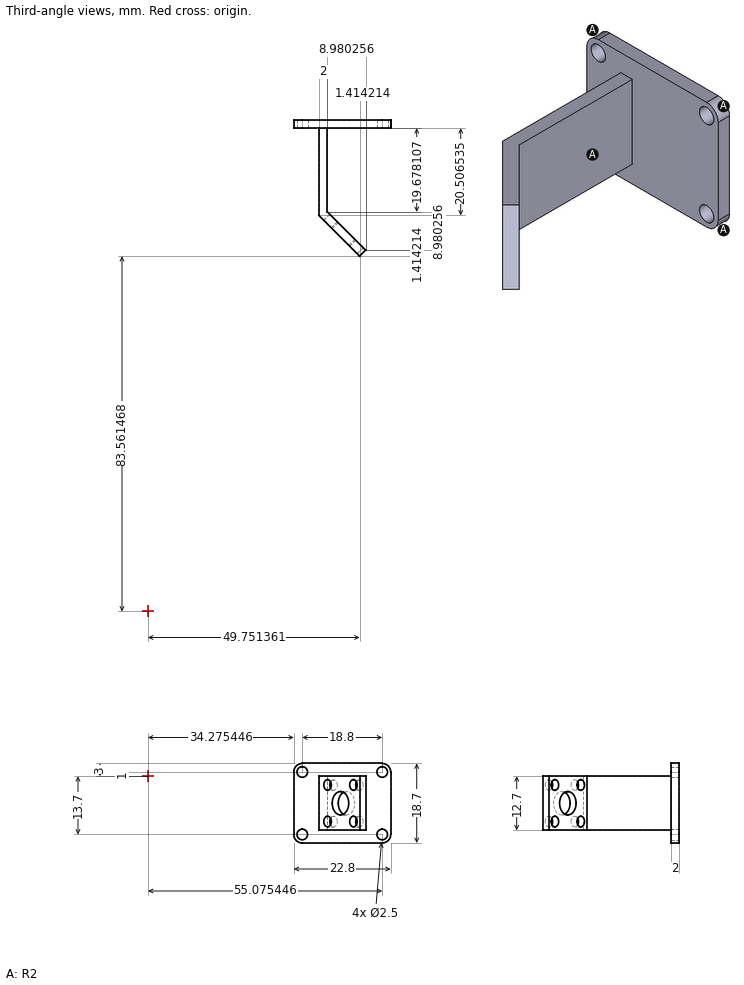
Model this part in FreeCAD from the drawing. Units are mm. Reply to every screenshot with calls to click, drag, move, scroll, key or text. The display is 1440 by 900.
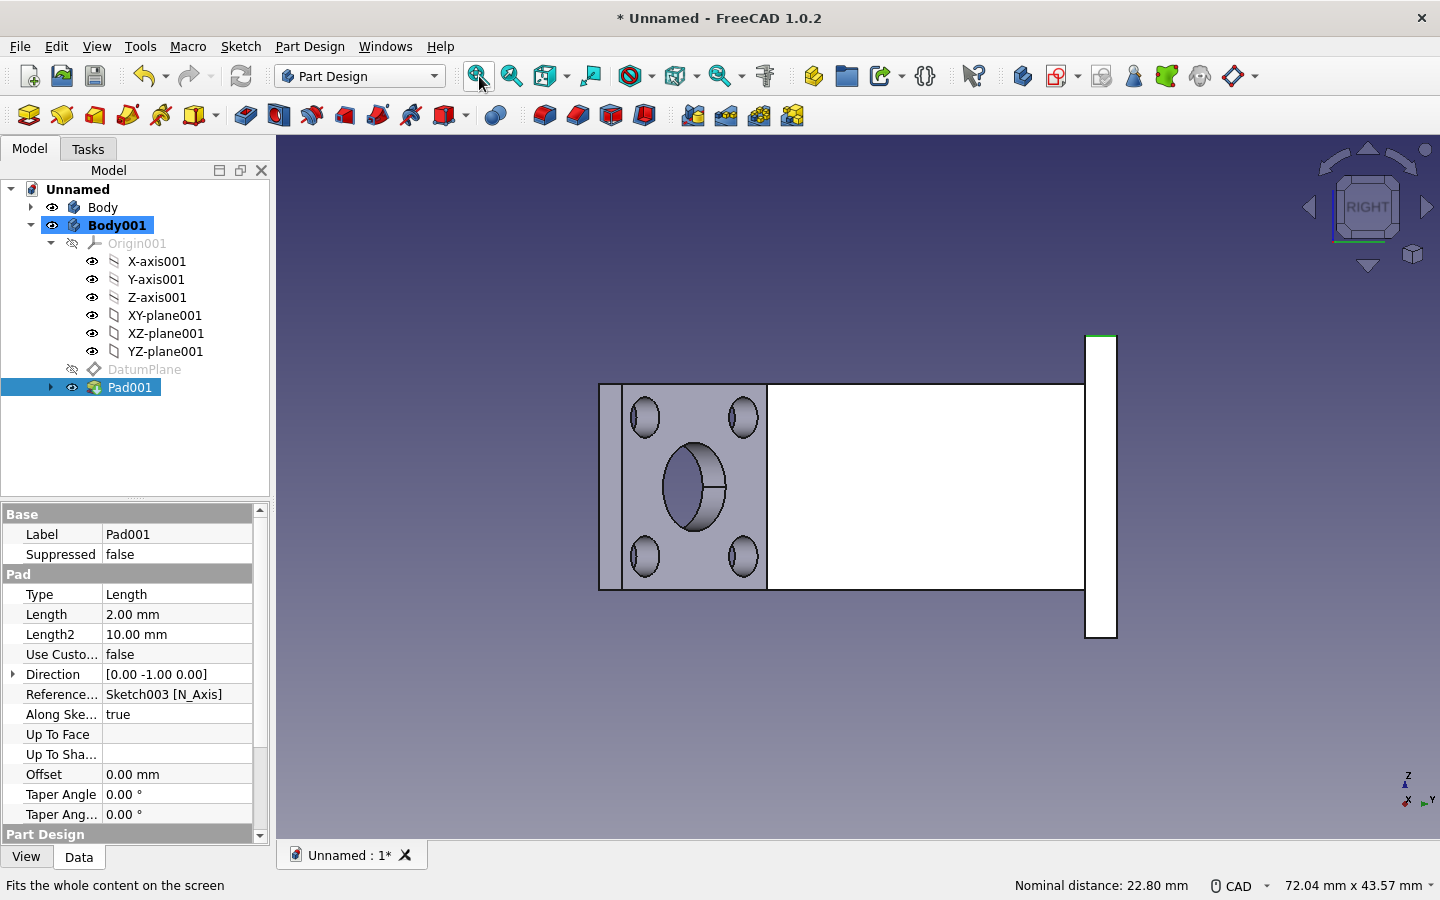
click(479, 76)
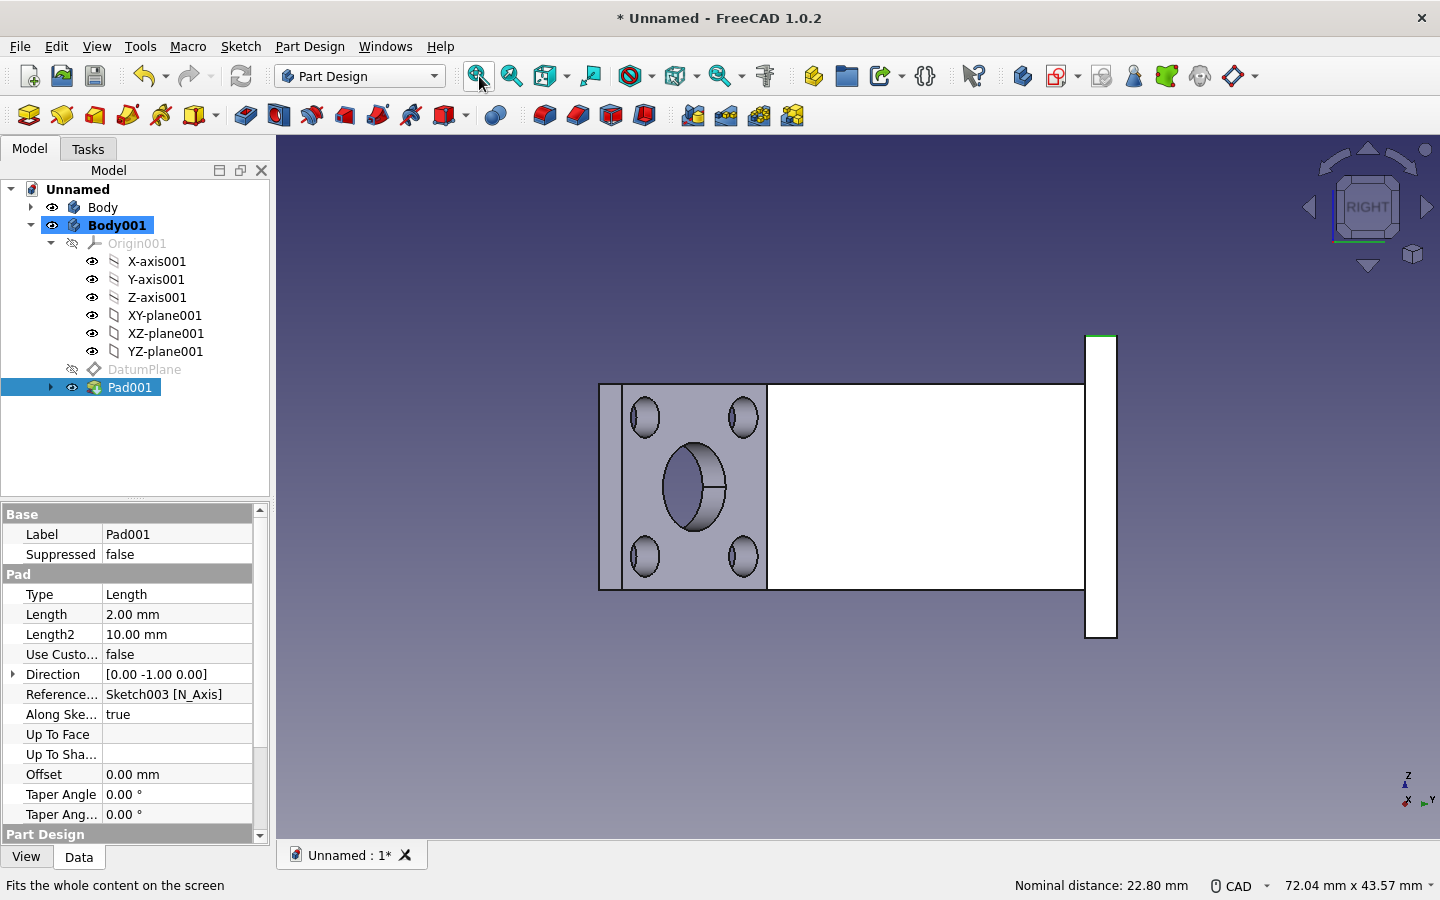
click(1101, 637, ctrl)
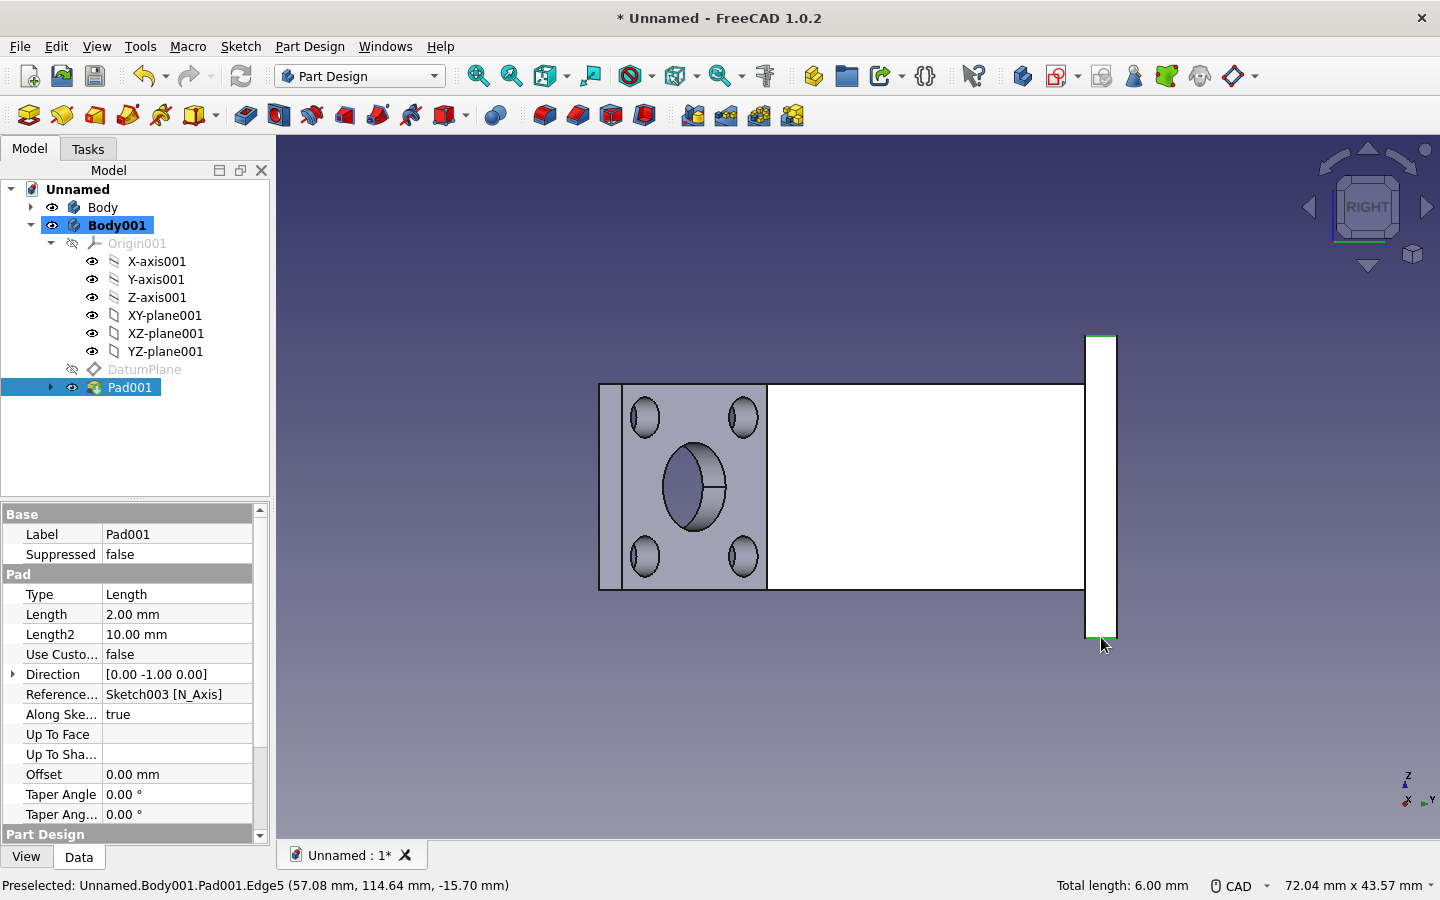
key(5)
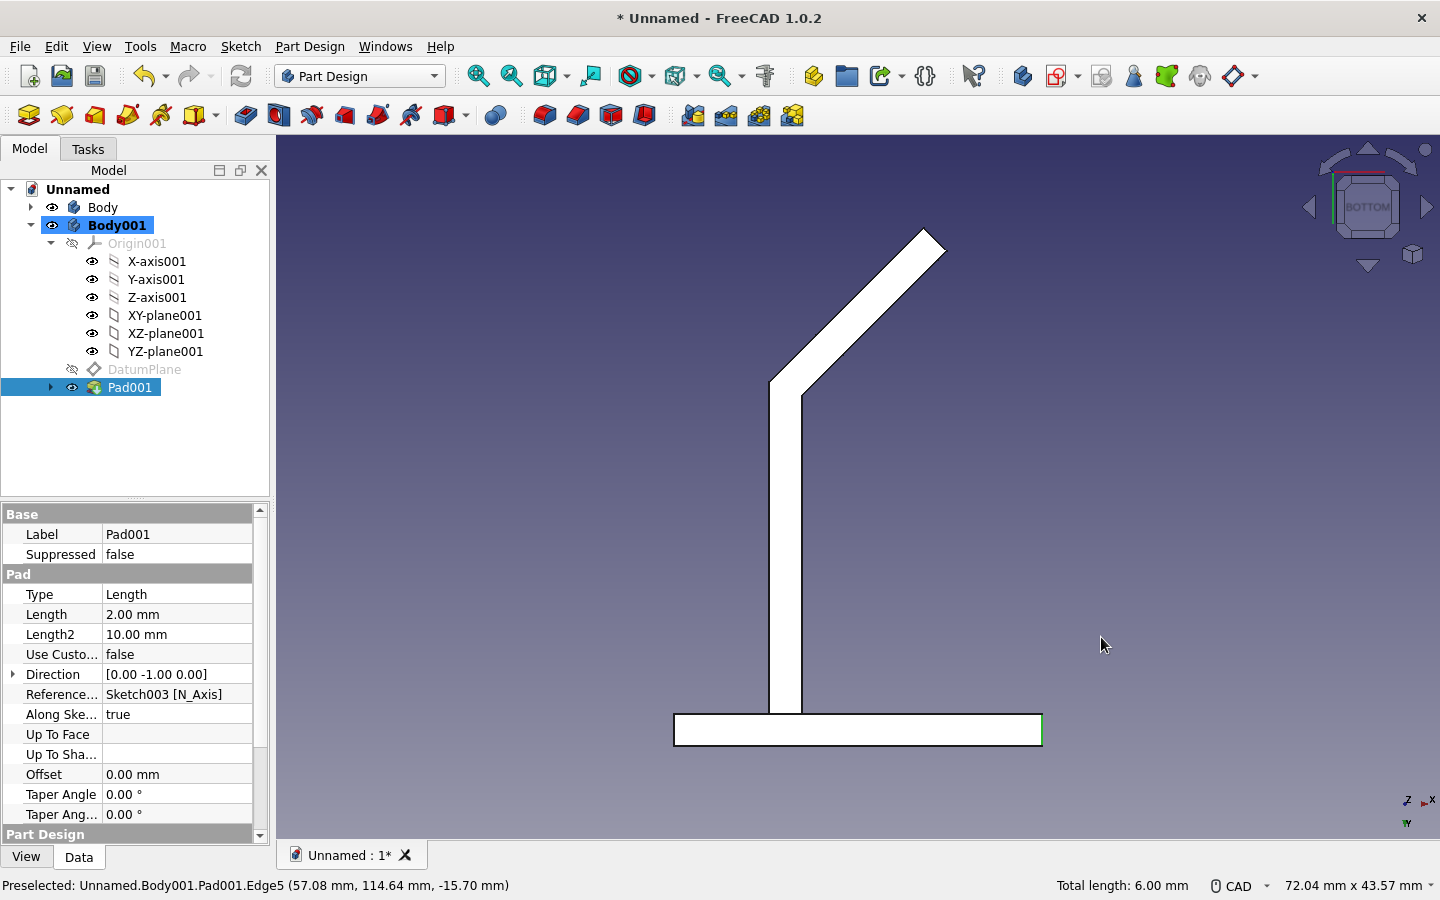
key(v)
key(f)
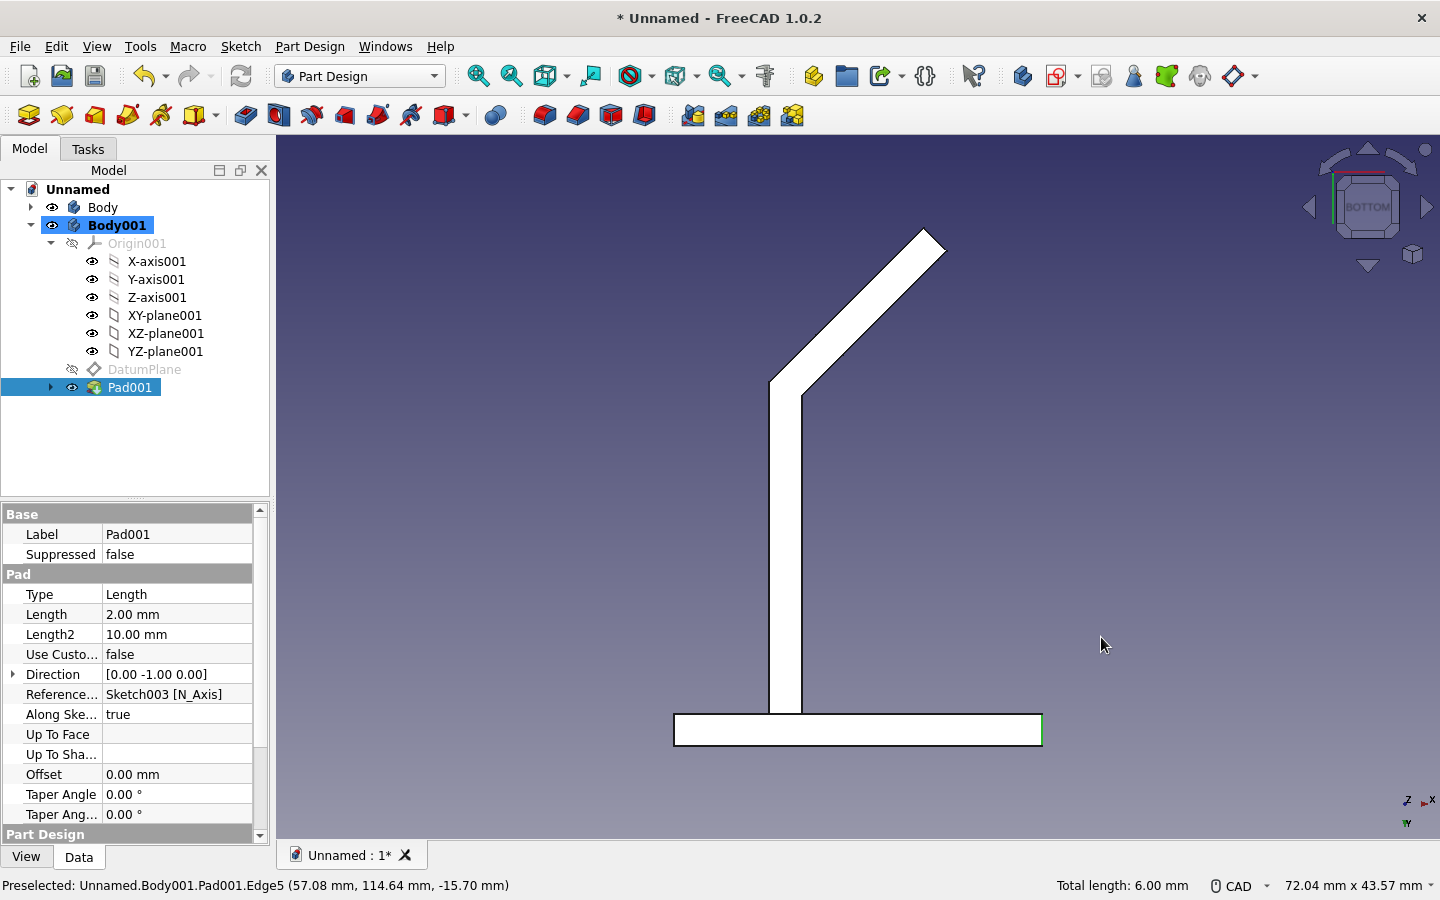
click(674, 729, ctrl)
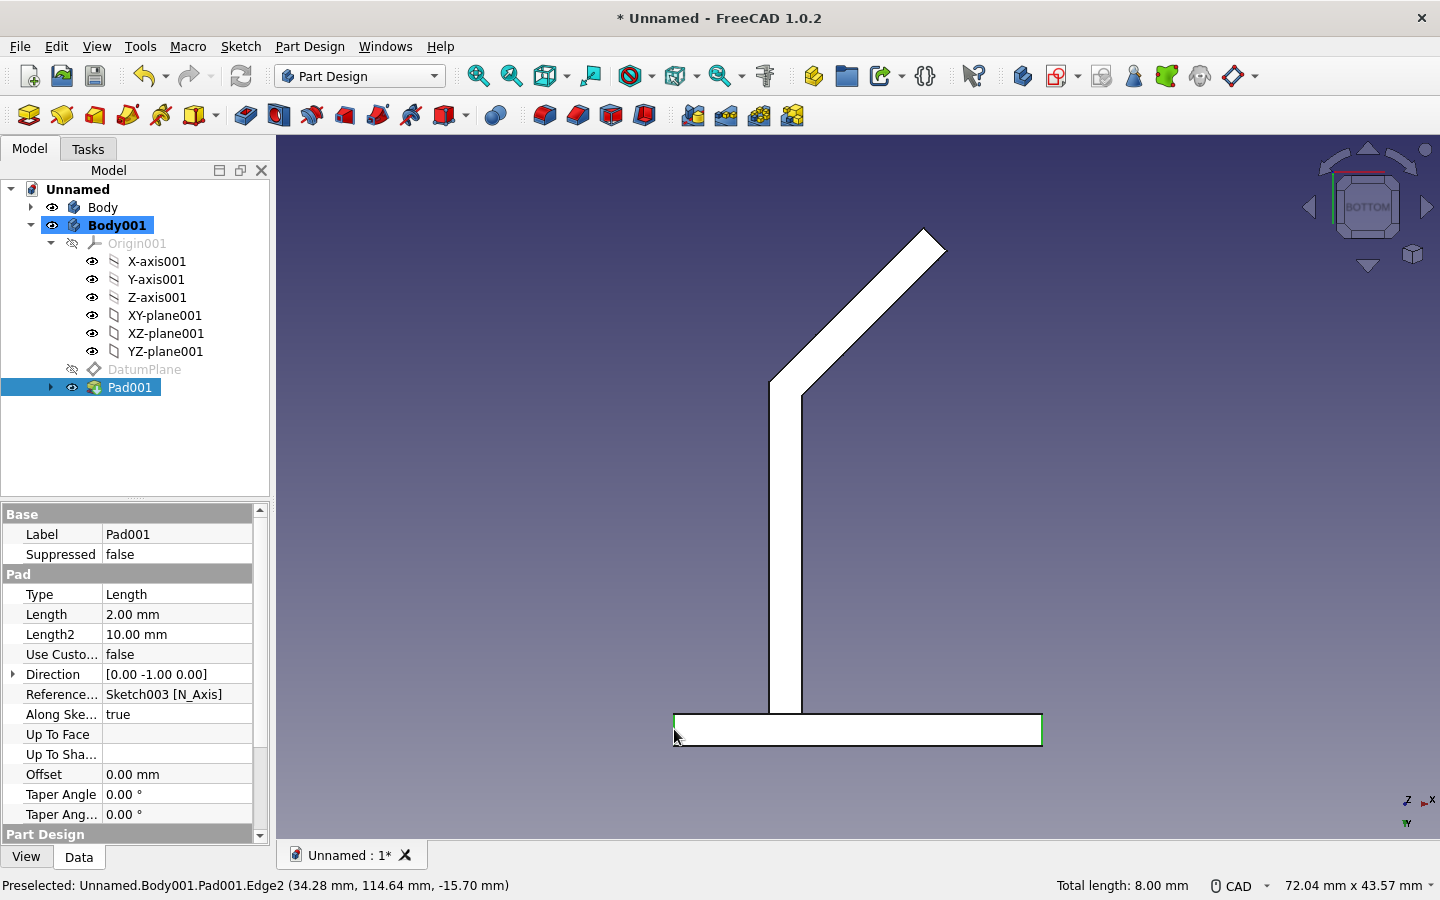
click(545, 116)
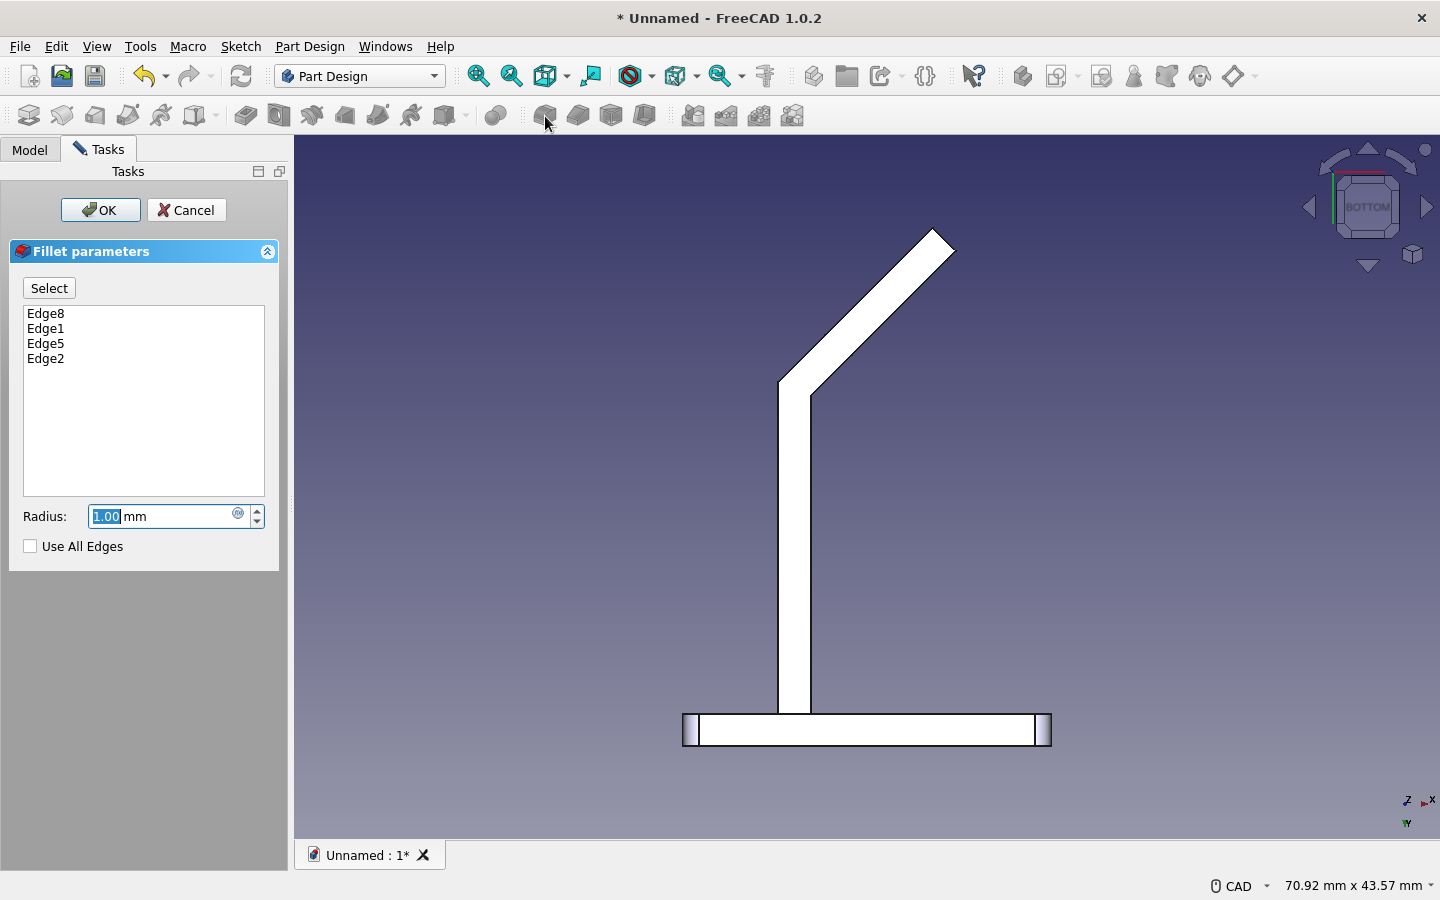
text(2)
key(Tab)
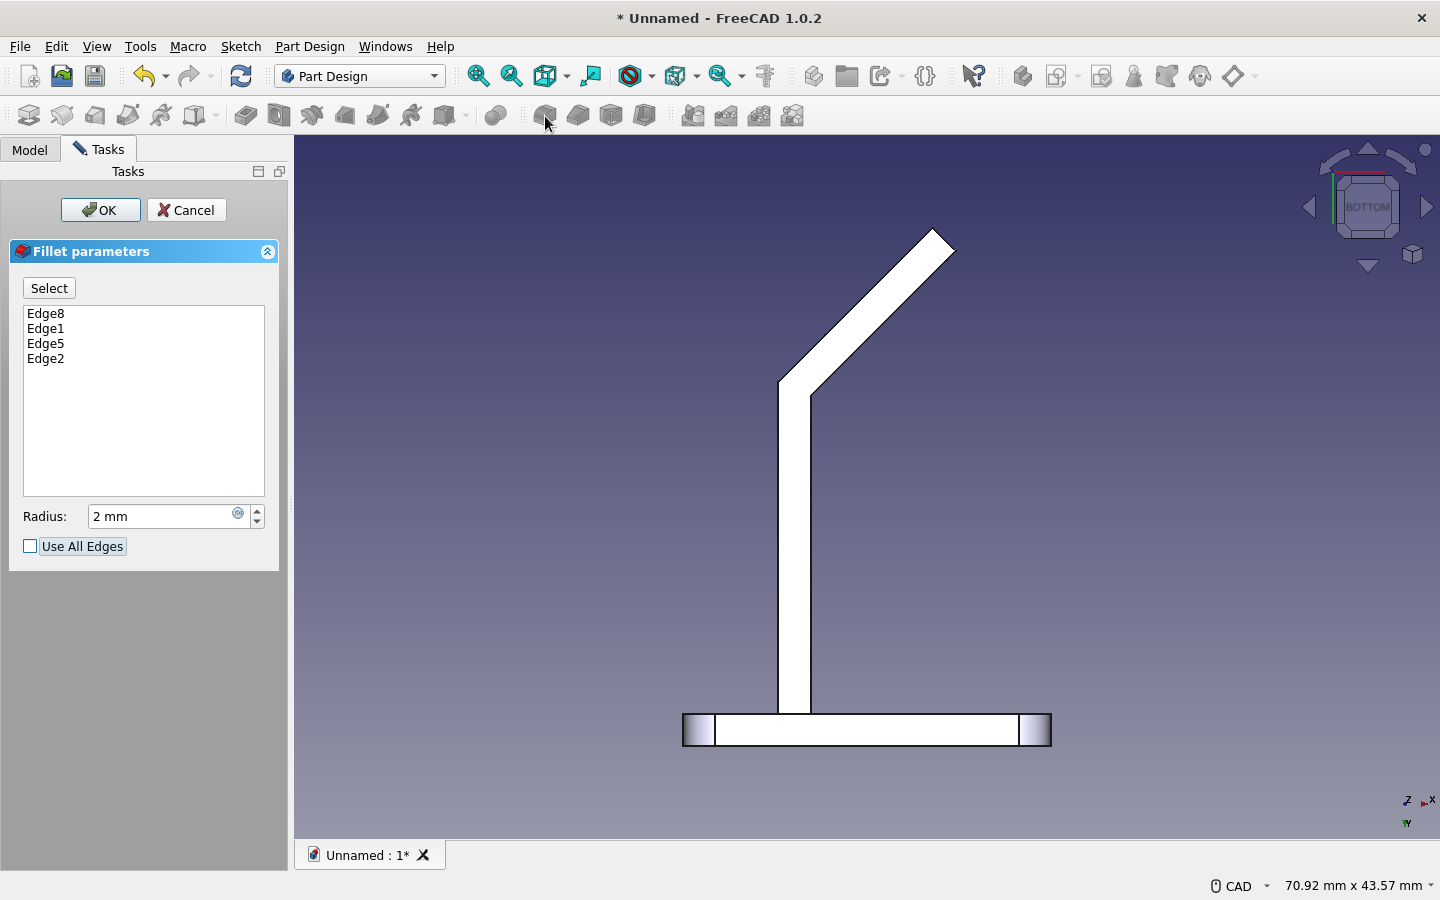
click(101, 210)